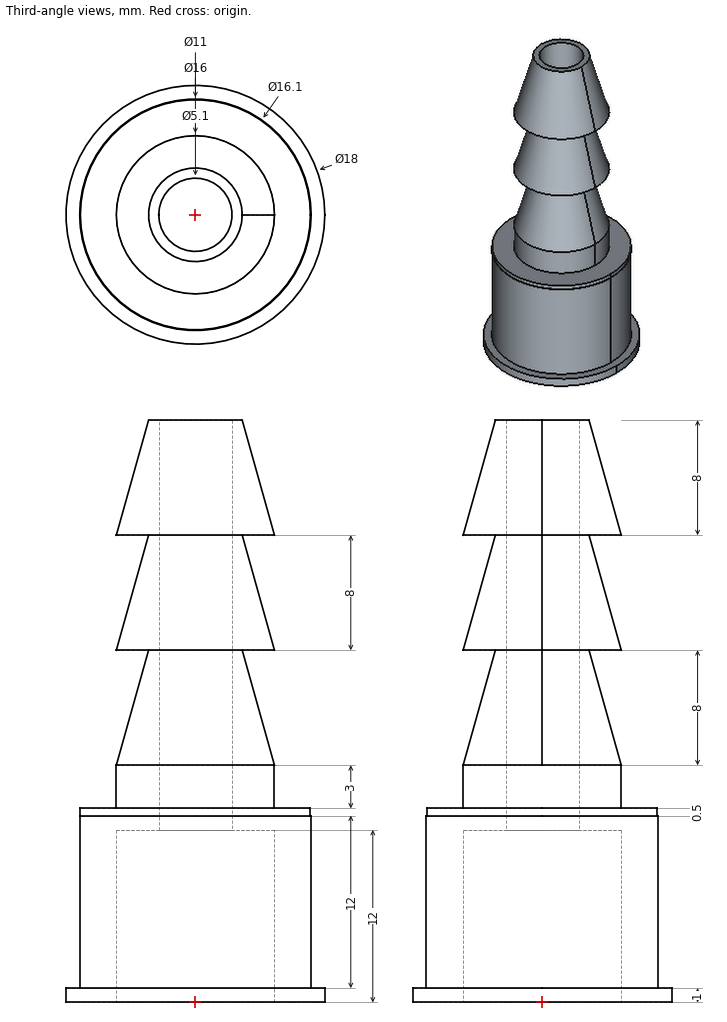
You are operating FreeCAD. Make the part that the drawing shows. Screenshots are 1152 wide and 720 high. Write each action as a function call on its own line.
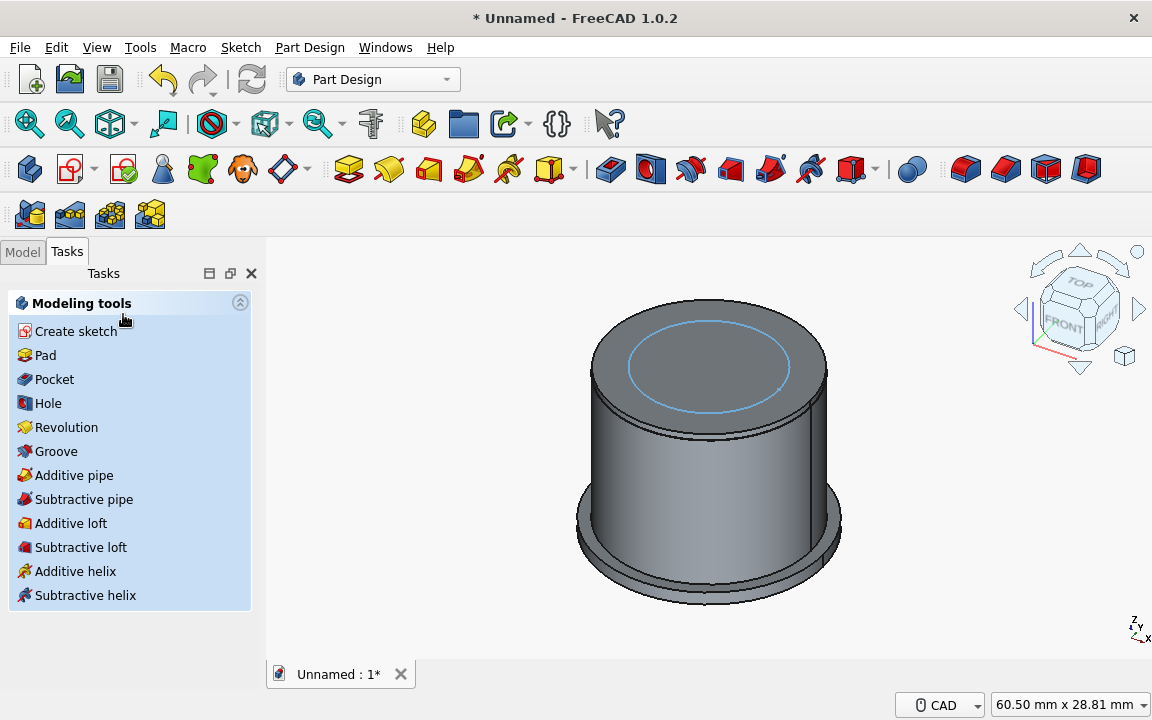
click(350, 170)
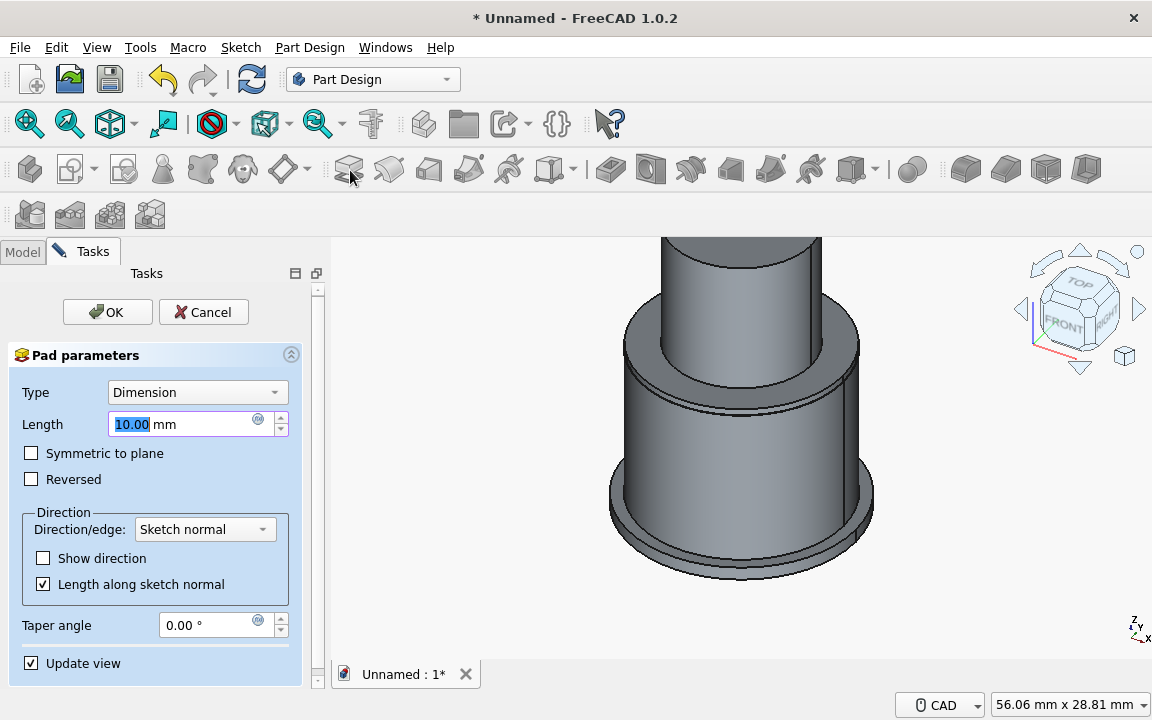
text(3)
key(Tab)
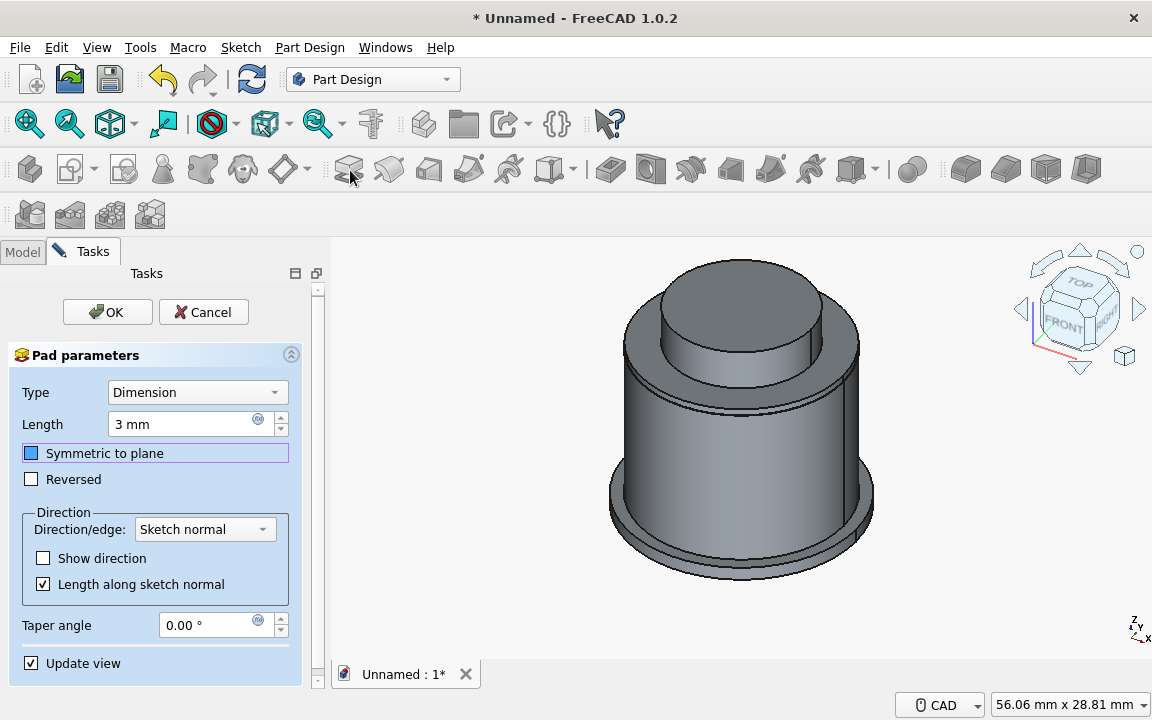
click(108, 312)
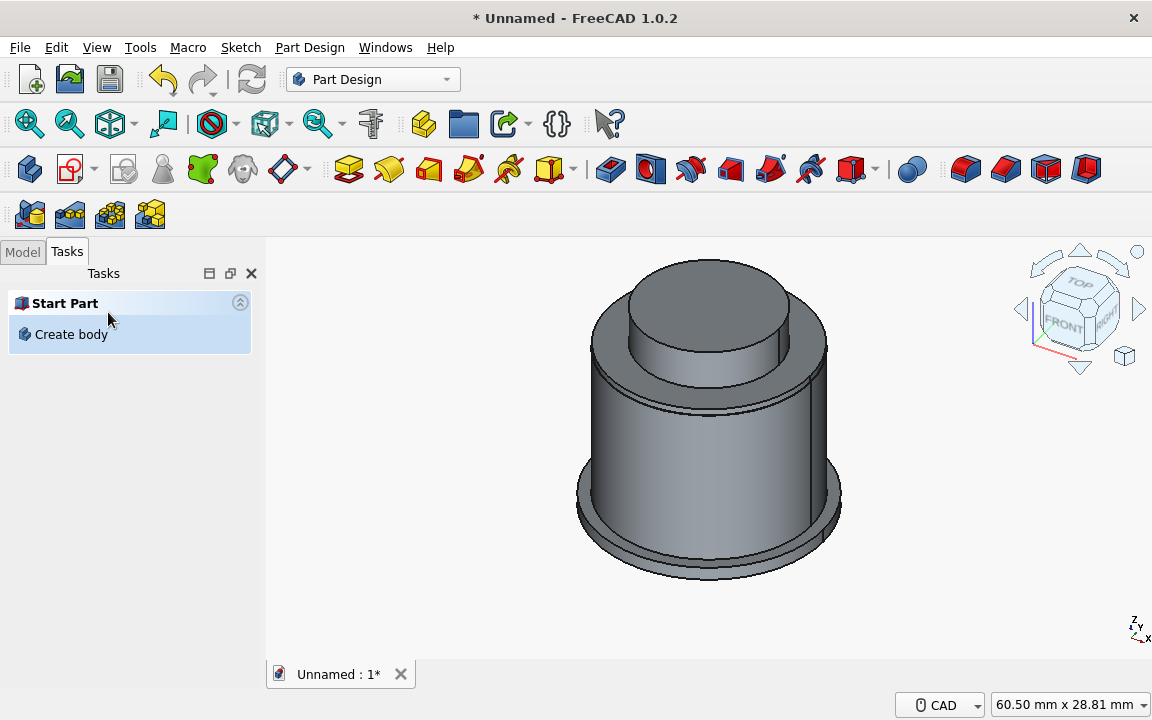
key(v)
key(f)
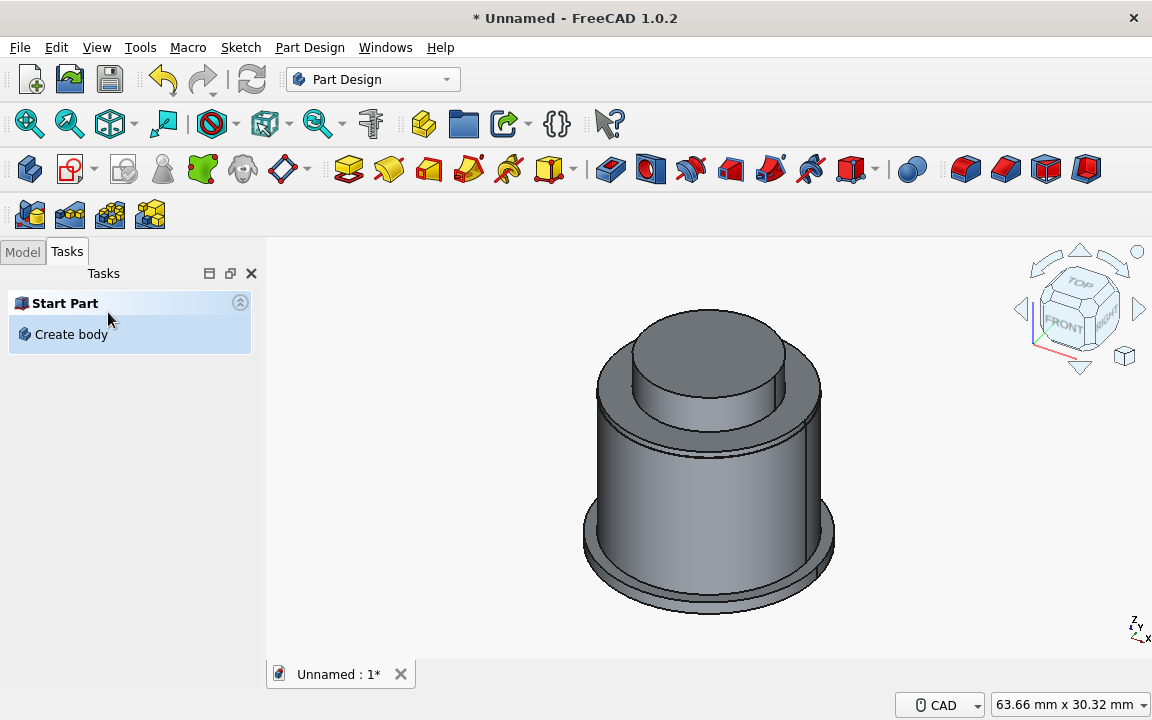
click(709, 353)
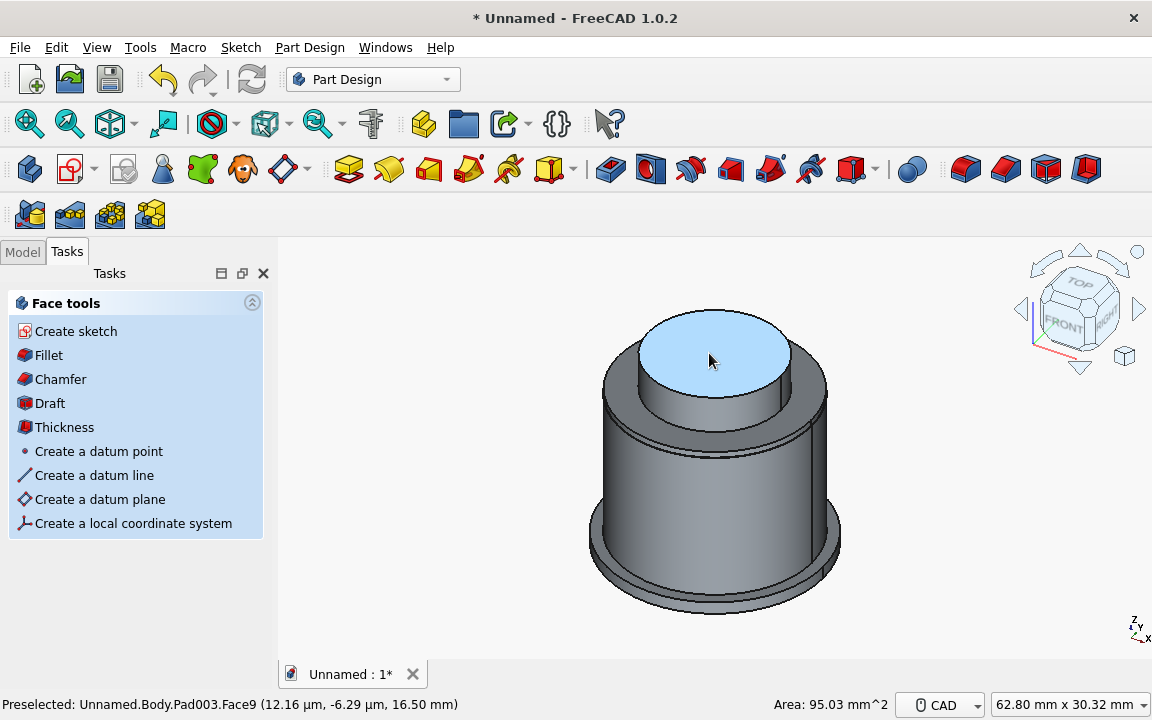
click(70, 170)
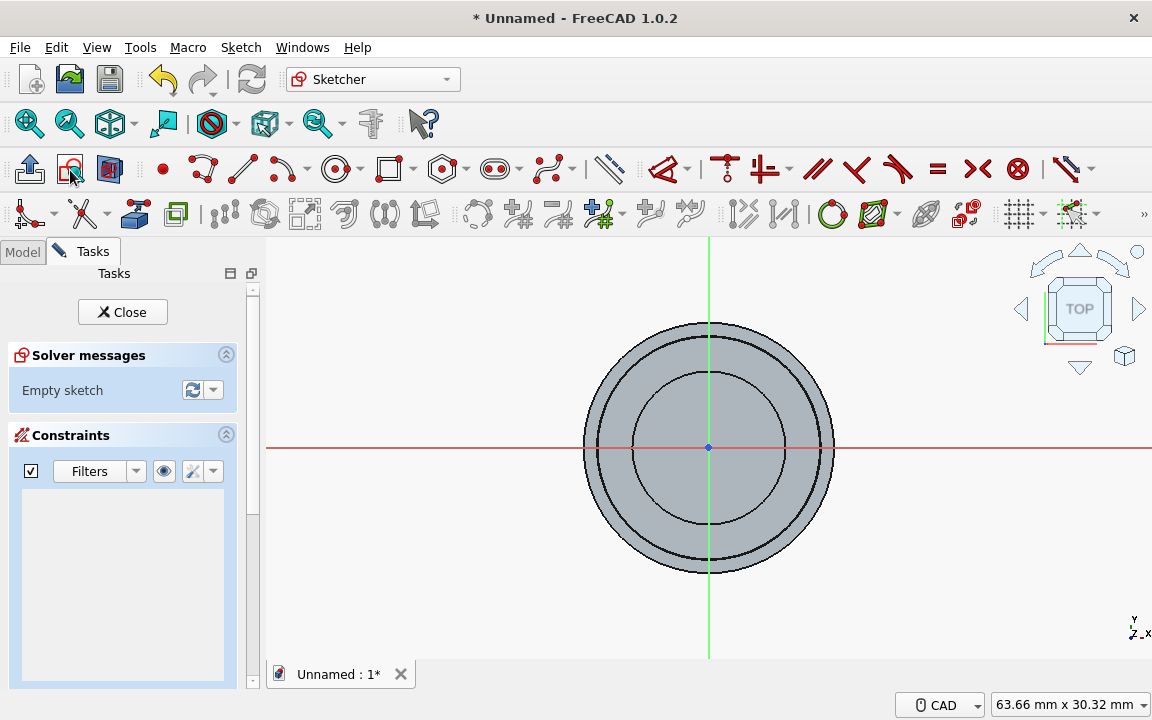
scroll(792, 448, up, 3)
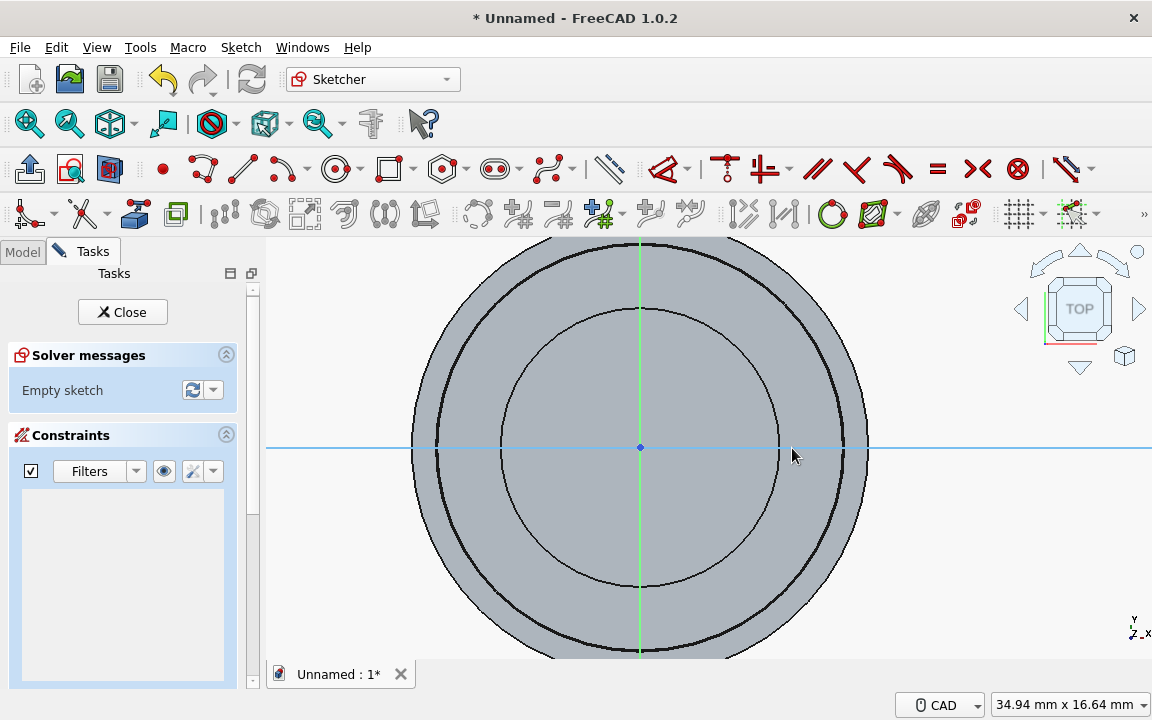
key(g)
key(c)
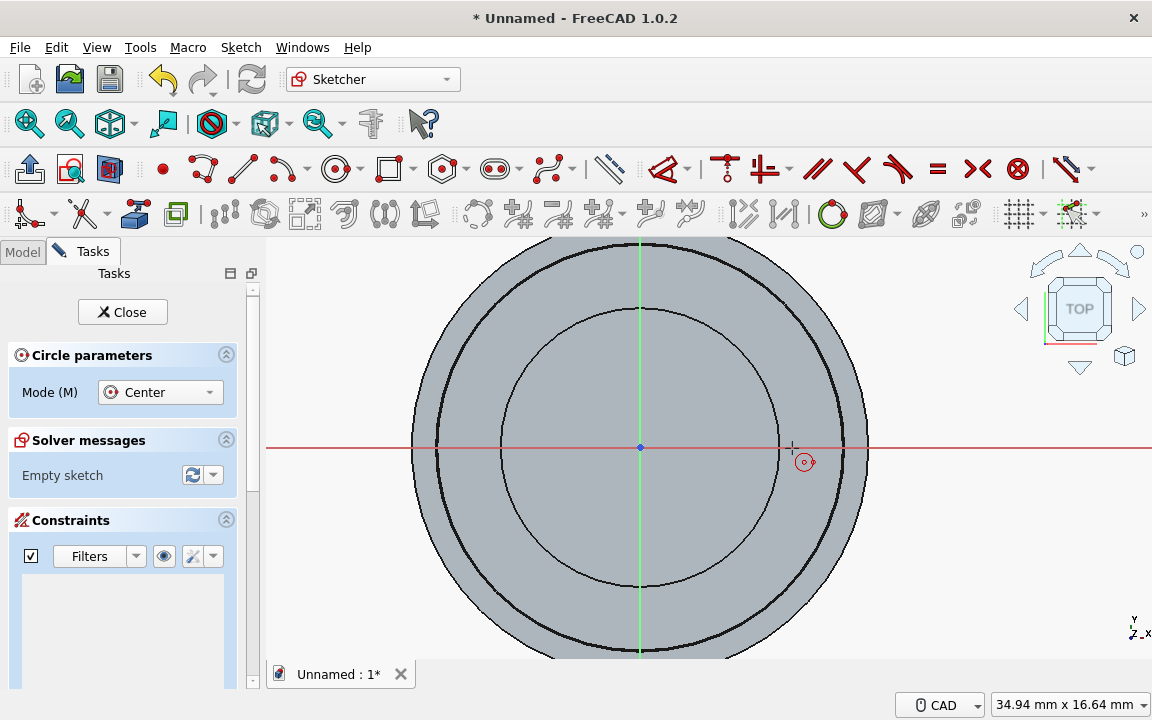
click(640, 448)
click(739, 349)
key(Escape)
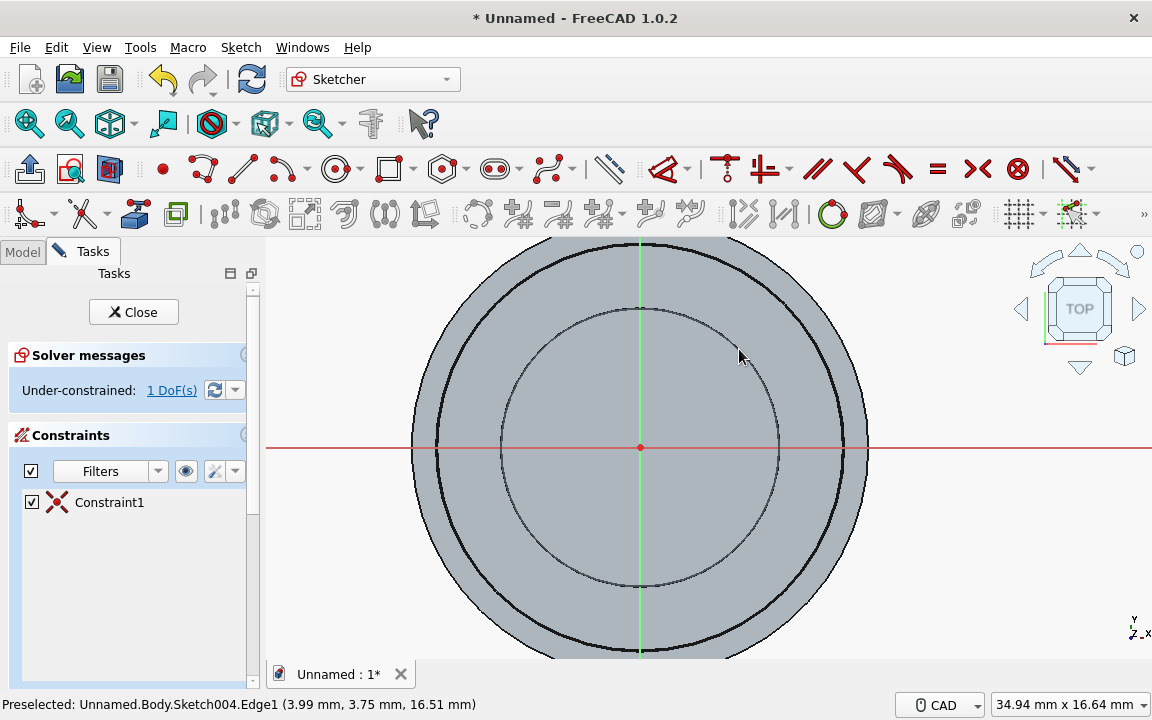
key(d)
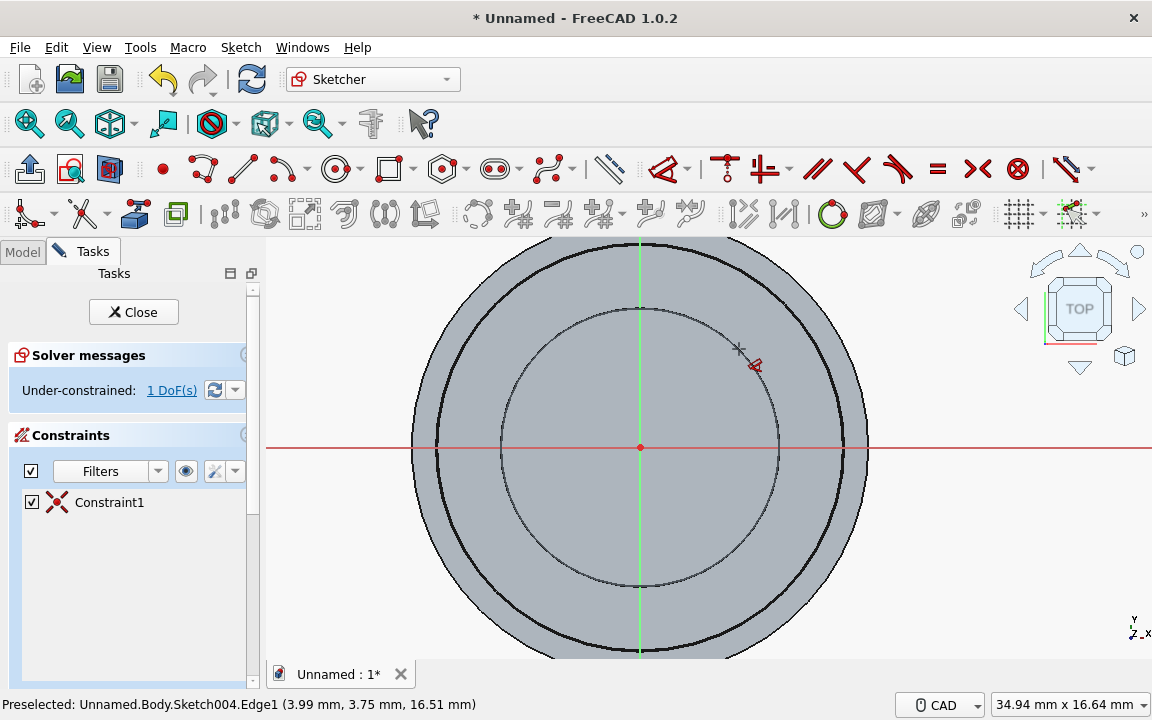
click(738, 349)
click(761, 326)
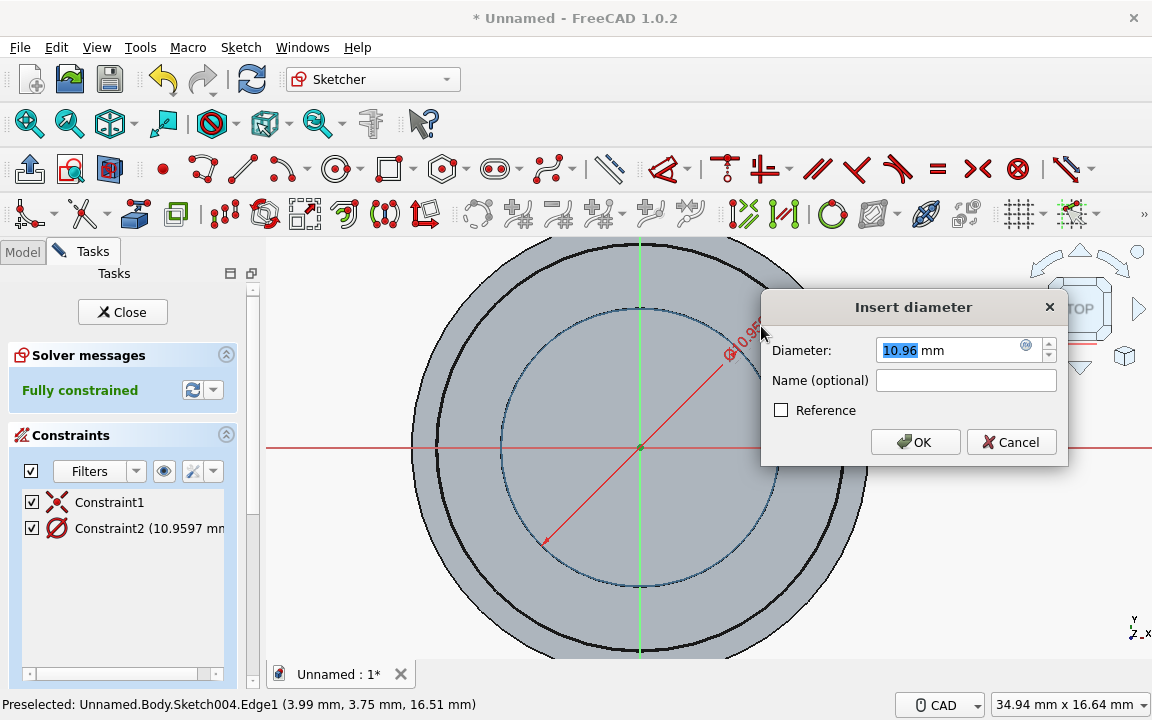
text(11)
key(Return)
key(Escape)